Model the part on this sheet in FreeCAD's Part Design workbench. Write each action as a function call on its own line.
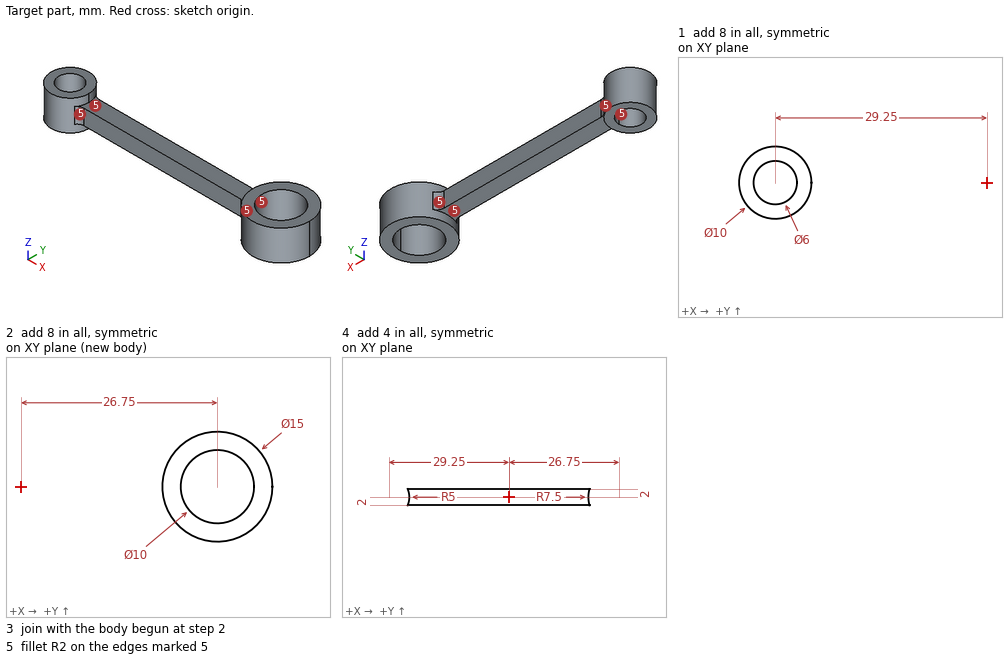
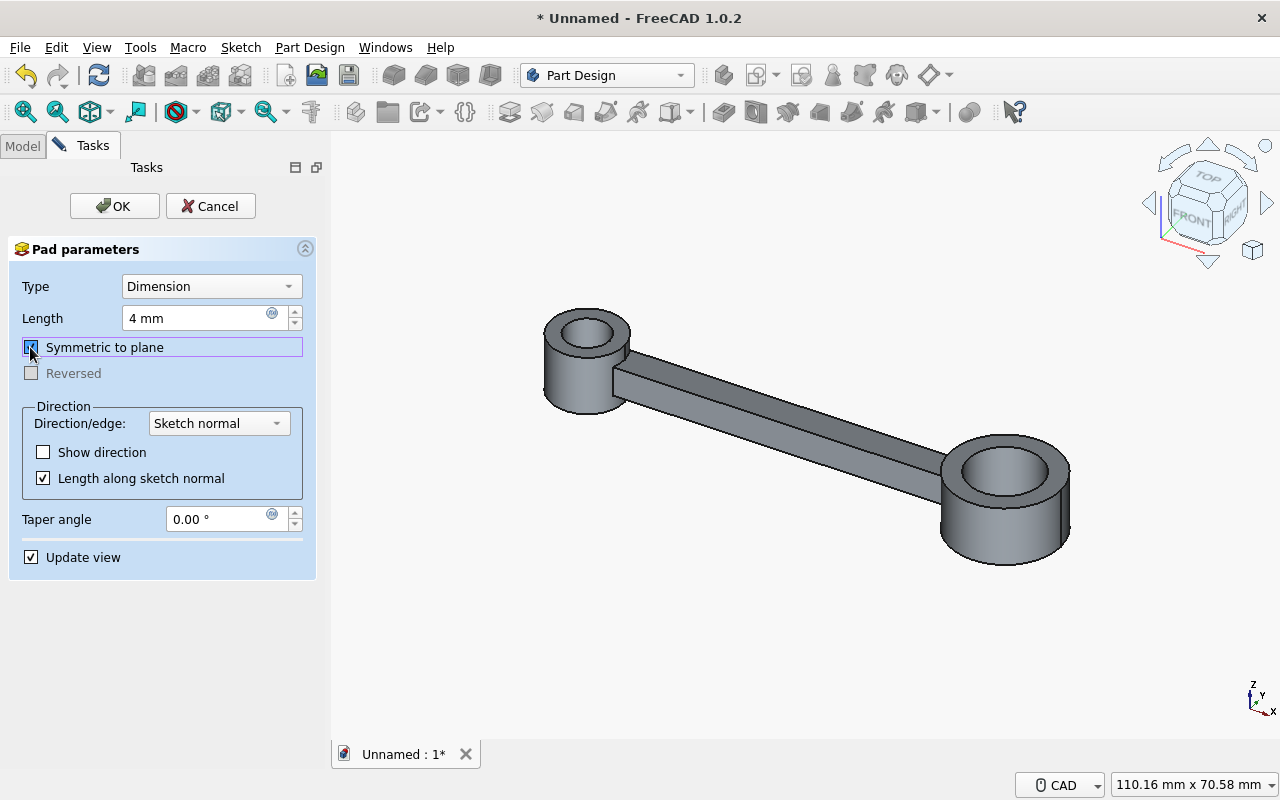
click(115, 206)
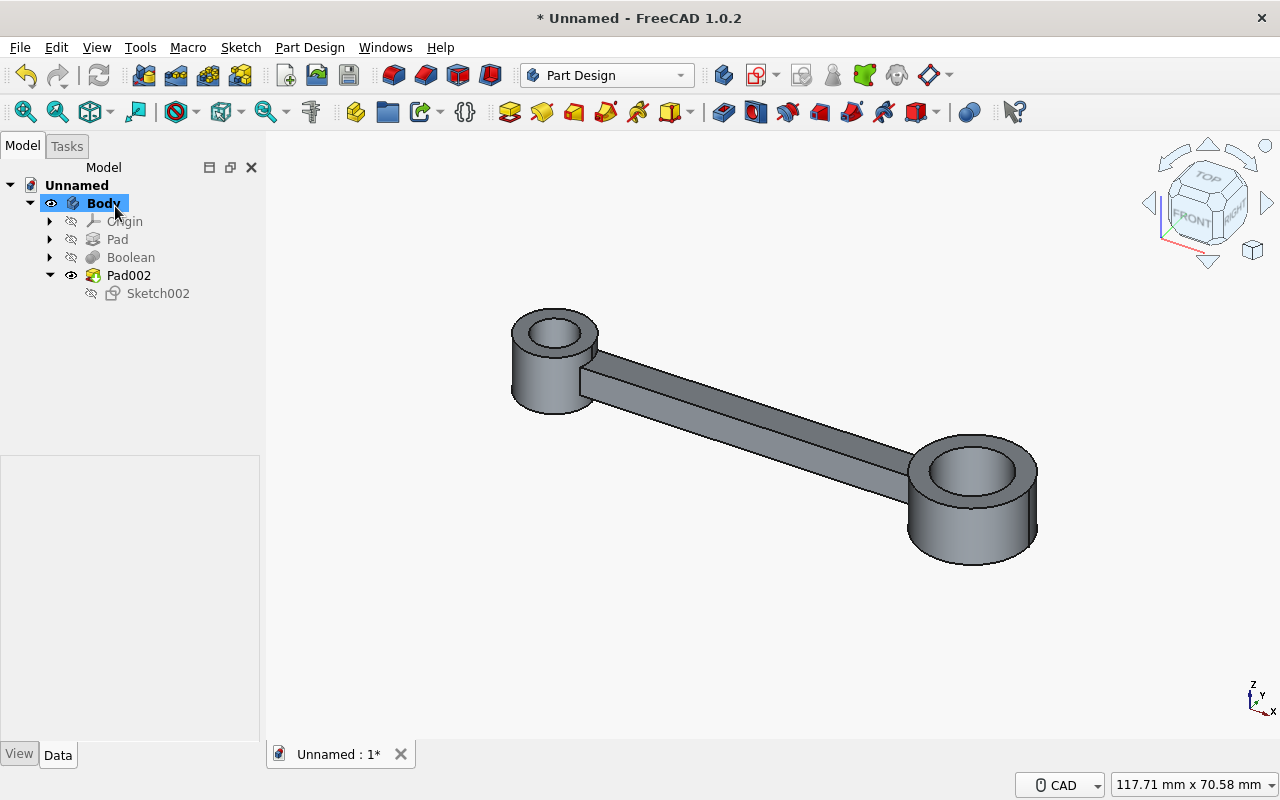
key(0)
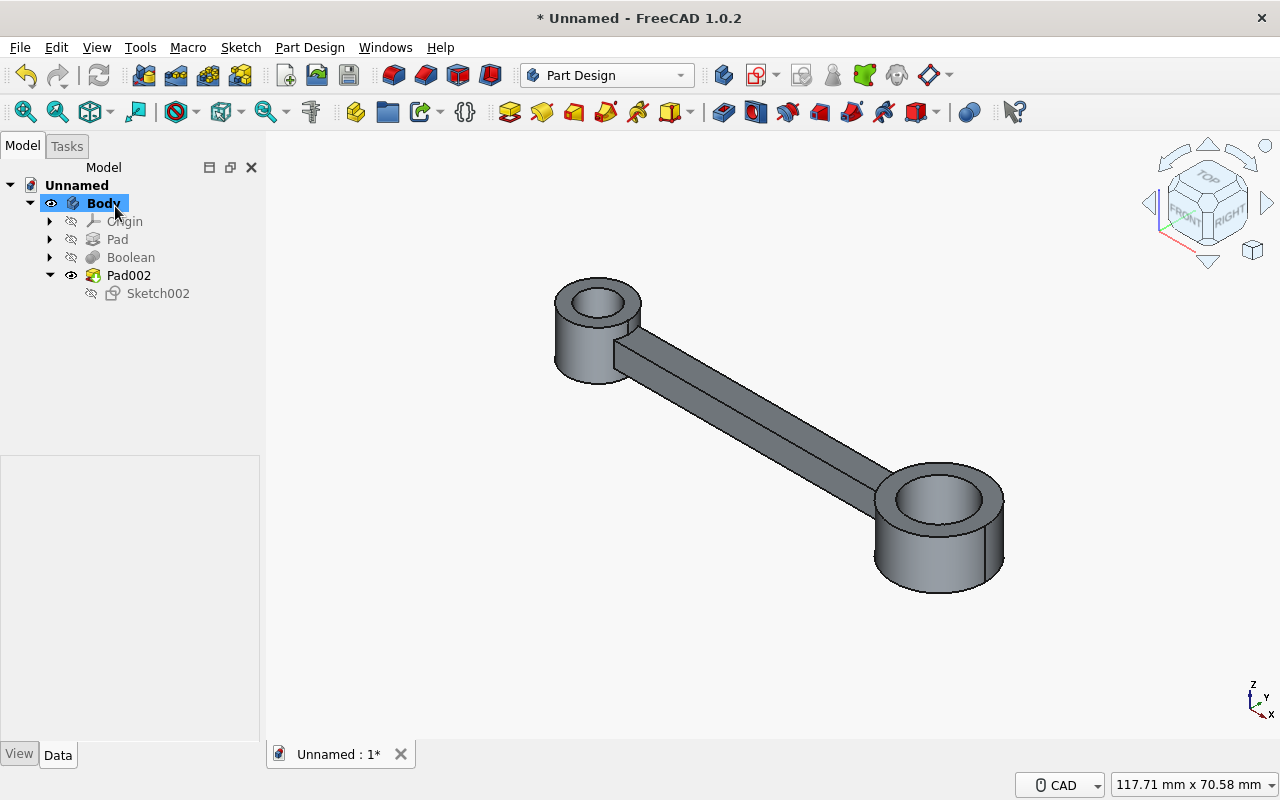
key(2)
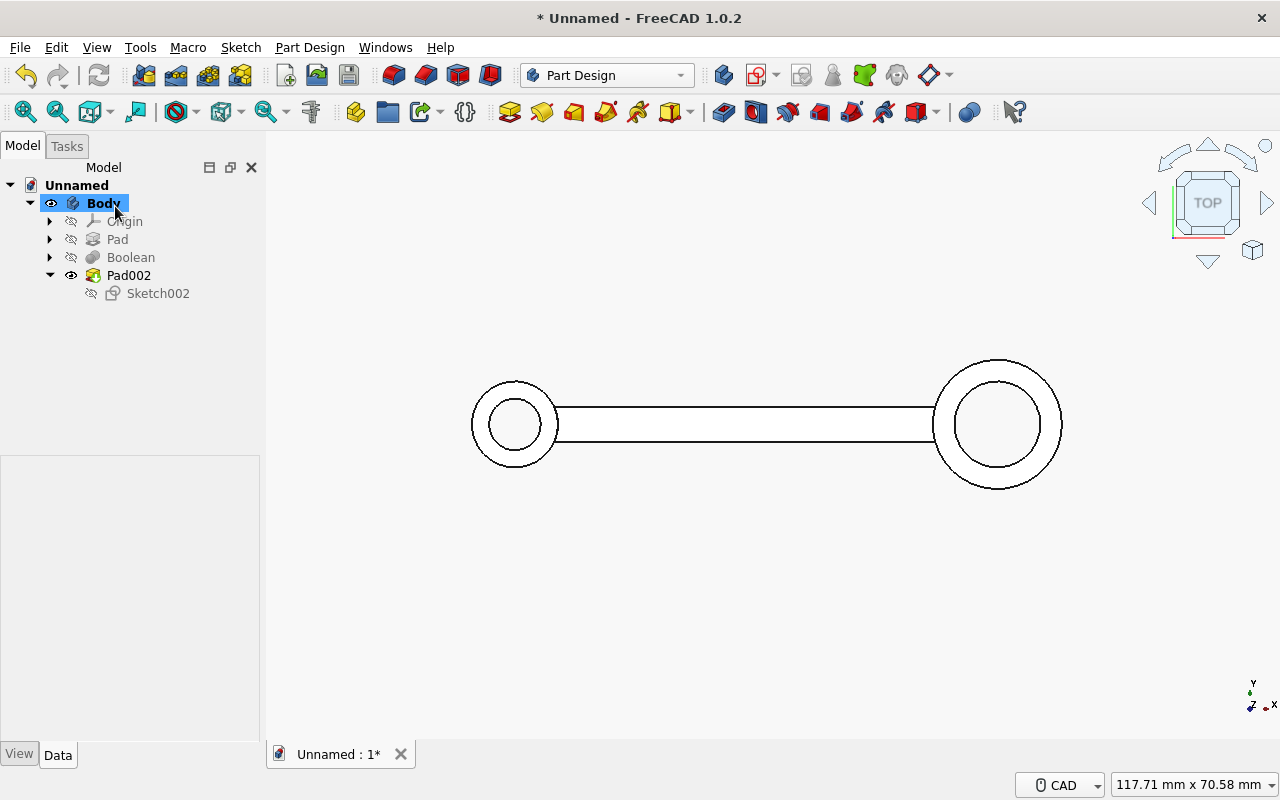
key(1)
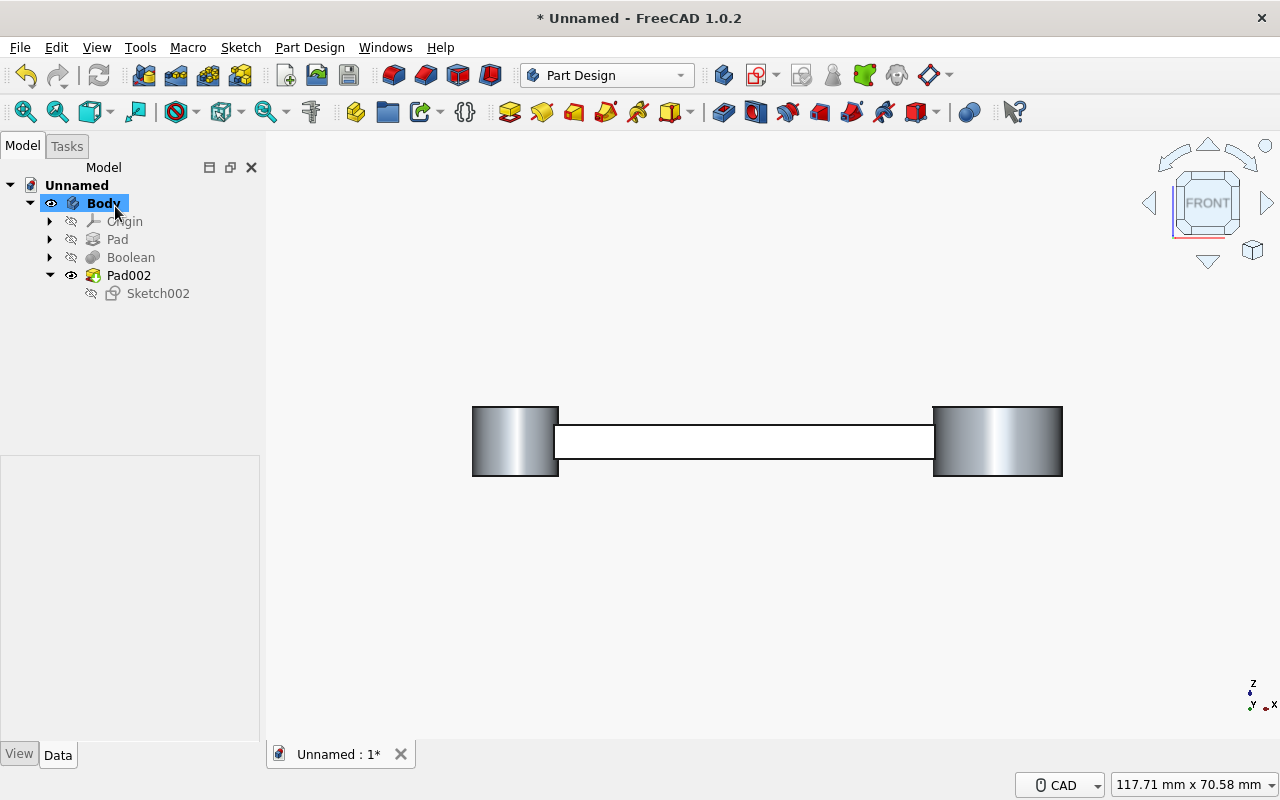
key(3)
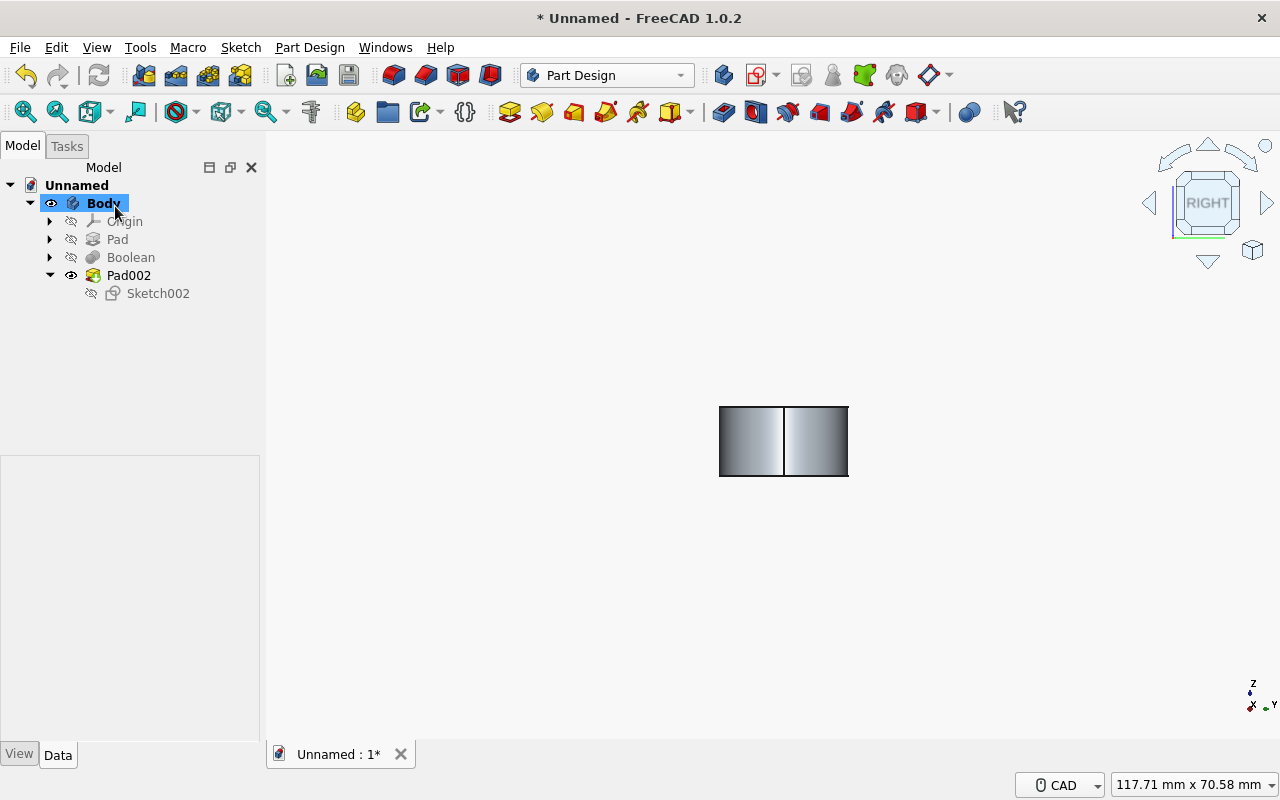
click(26, 112)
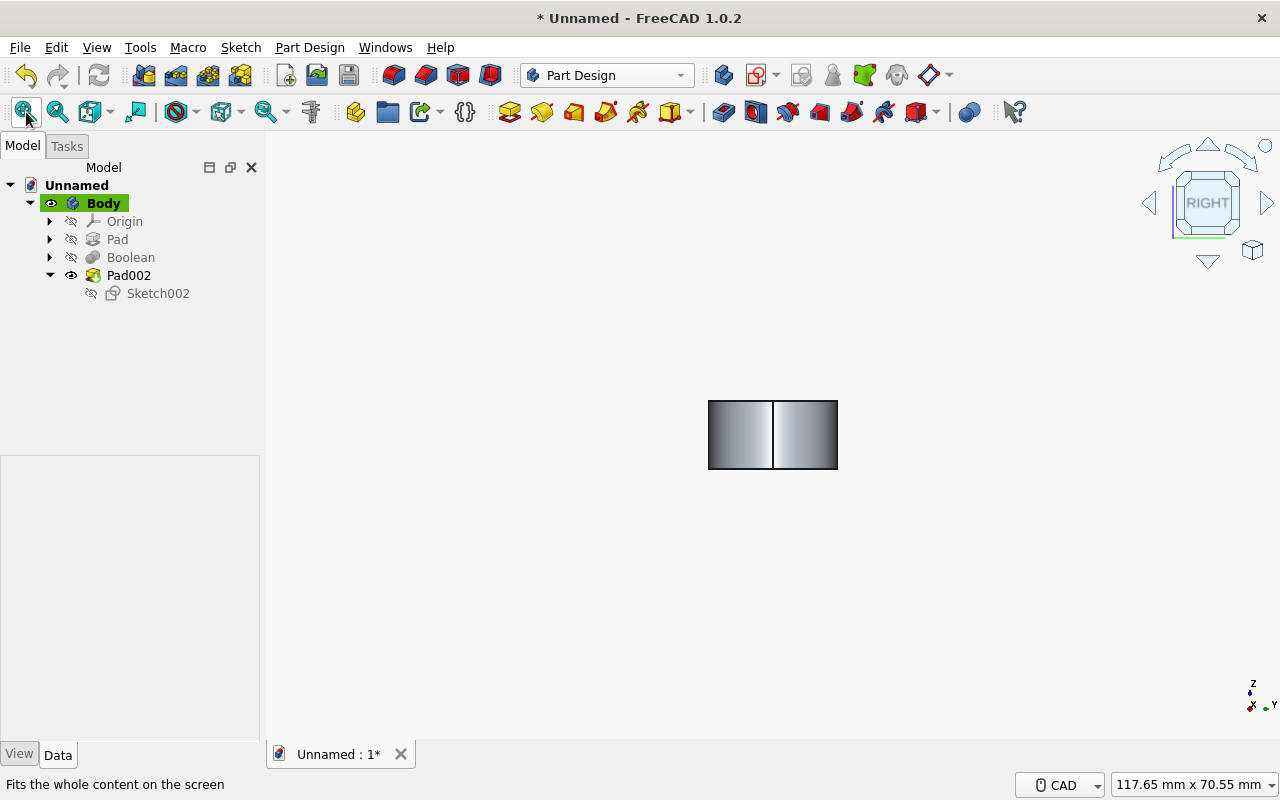
key(5)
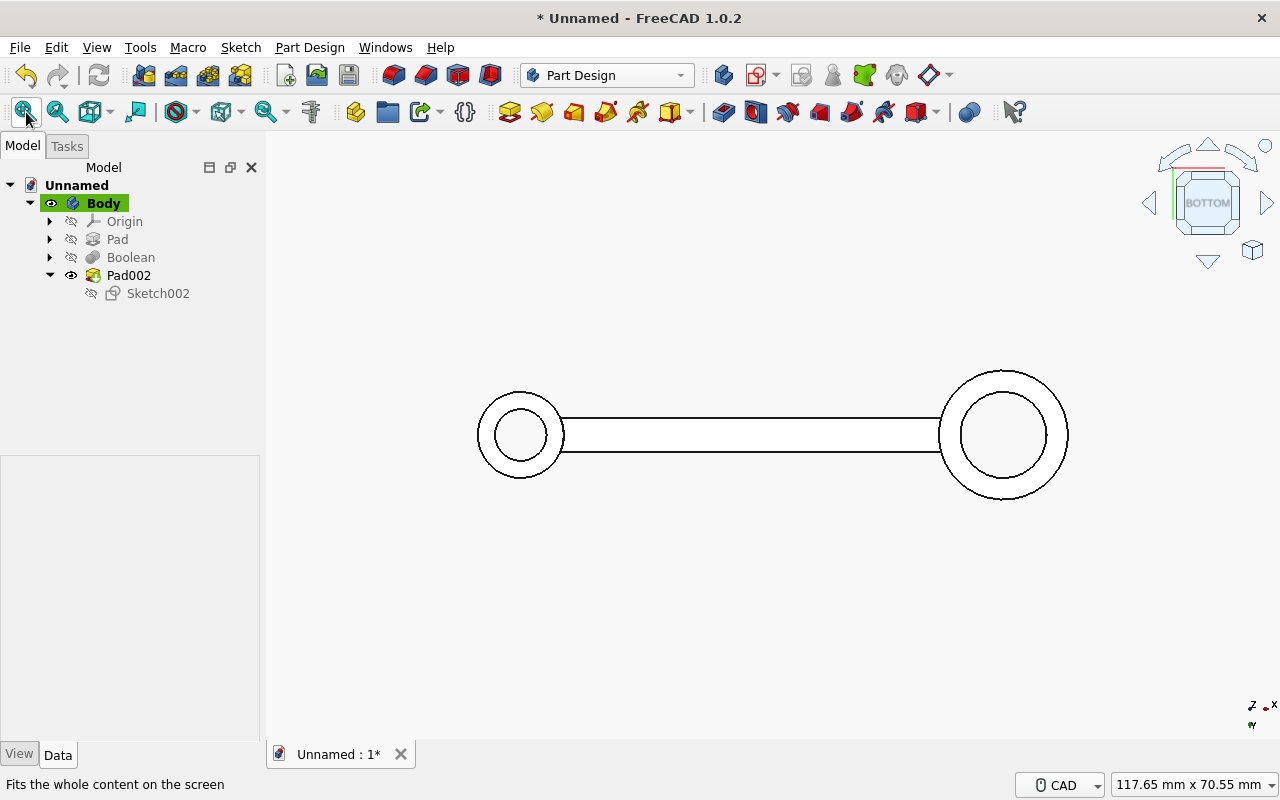
key(4)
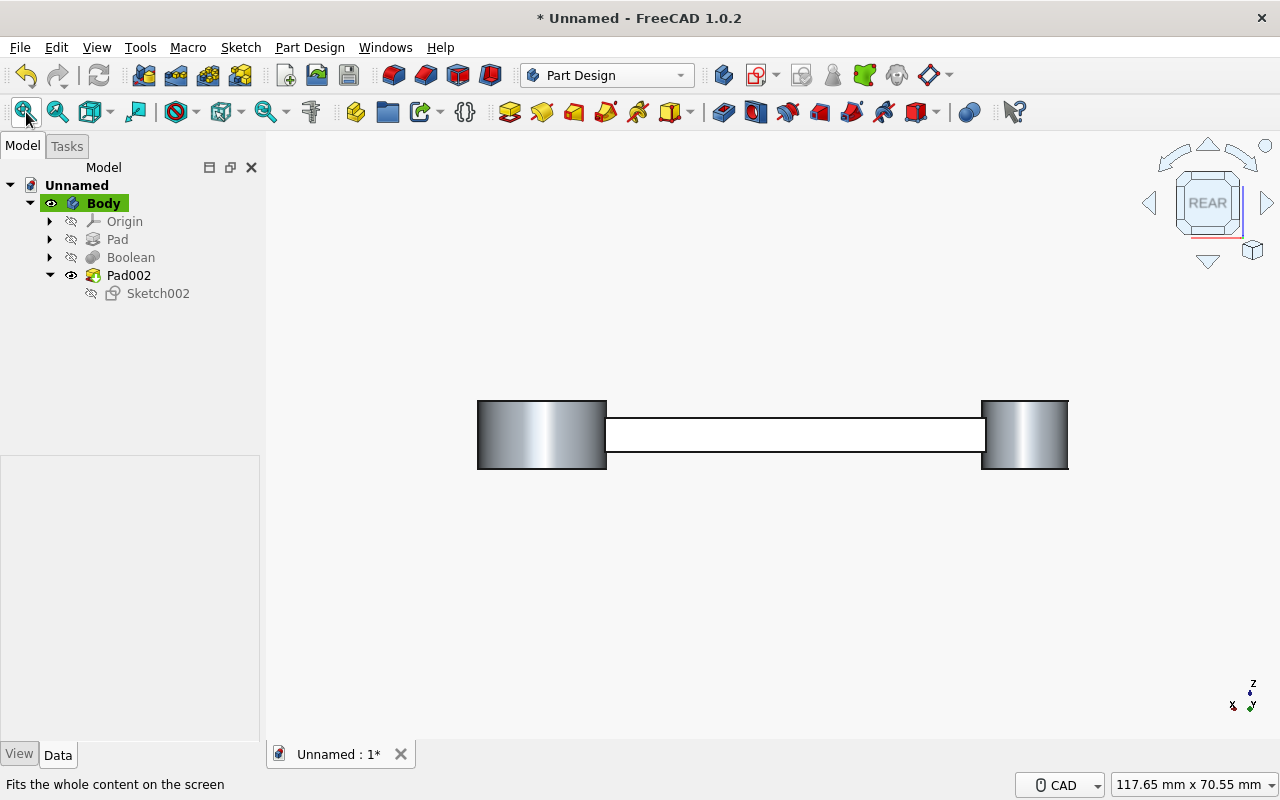
key(6)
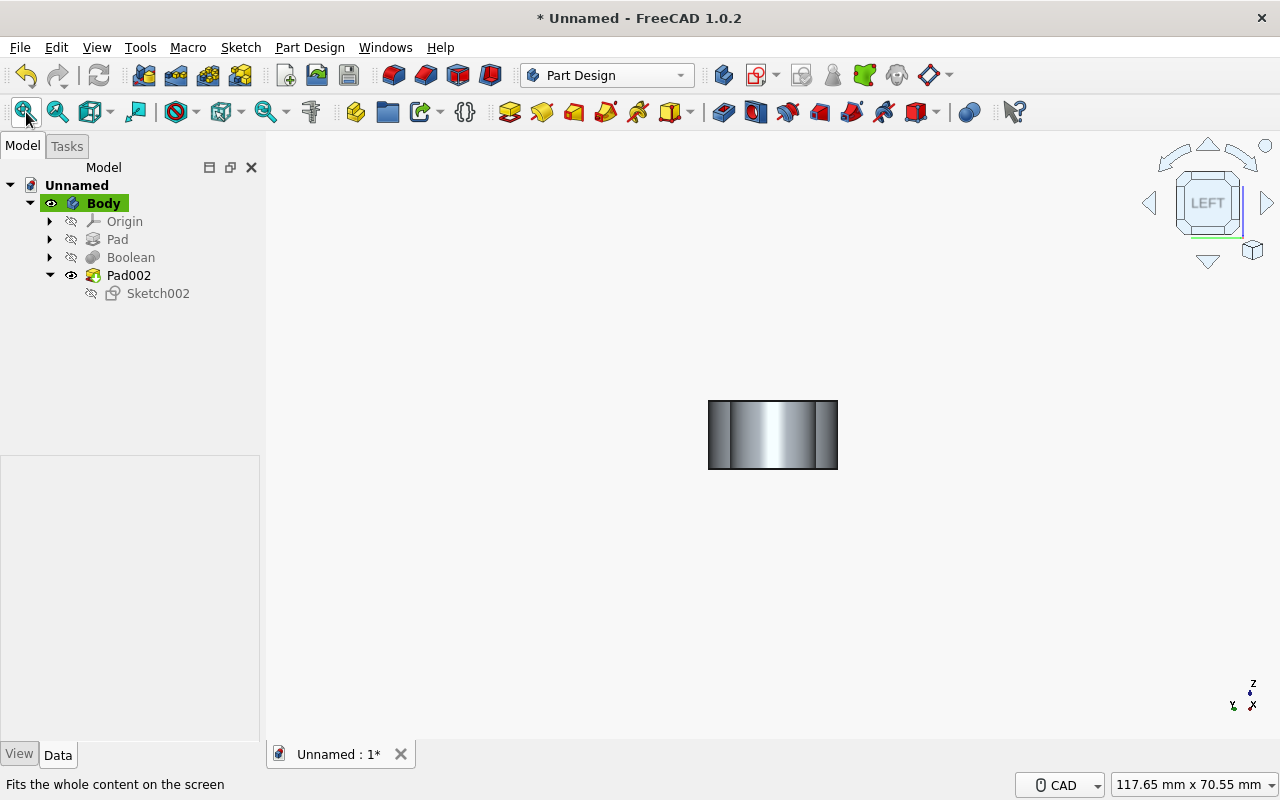
click(26, 112)